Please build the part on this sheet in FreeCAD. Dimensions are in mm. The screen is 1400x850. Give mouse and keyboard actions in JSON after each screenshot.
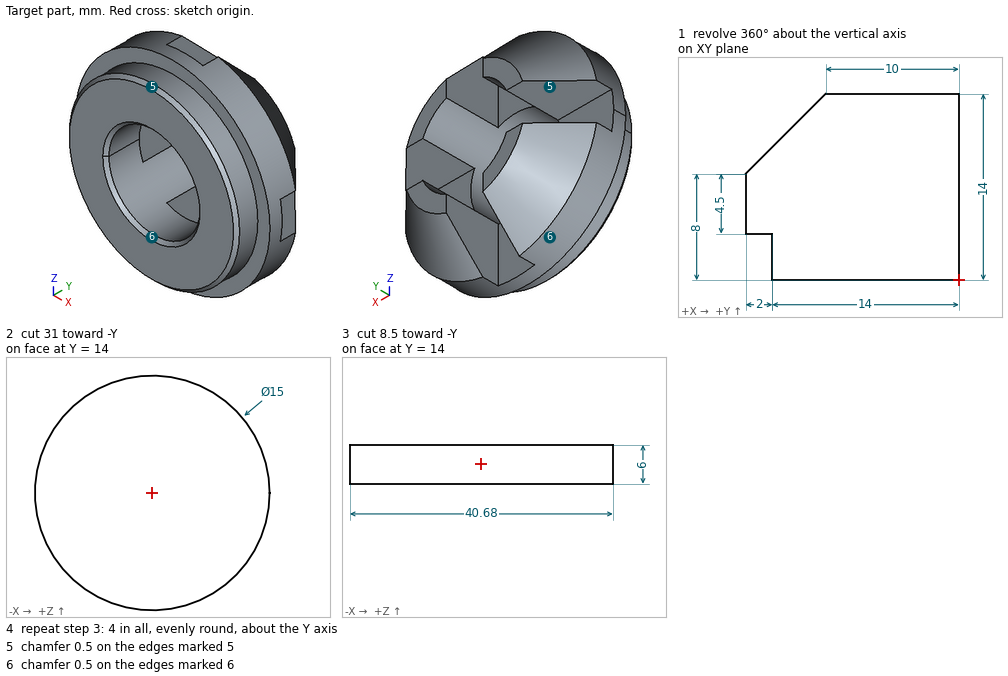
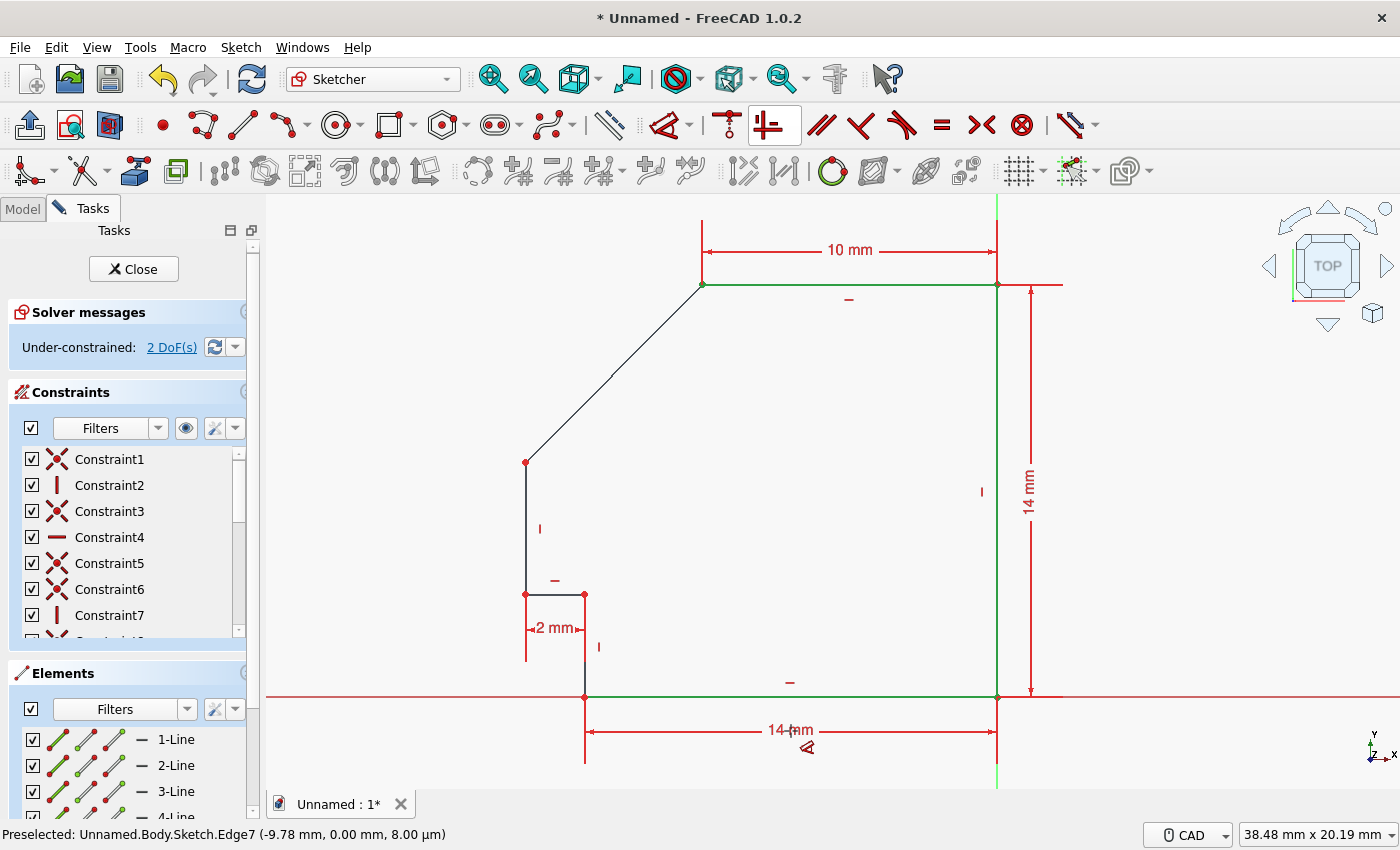
{"action": "left_click", "coordinate": [526, 463]}
{"action": "left_click", "coordinate": [1031, 580]}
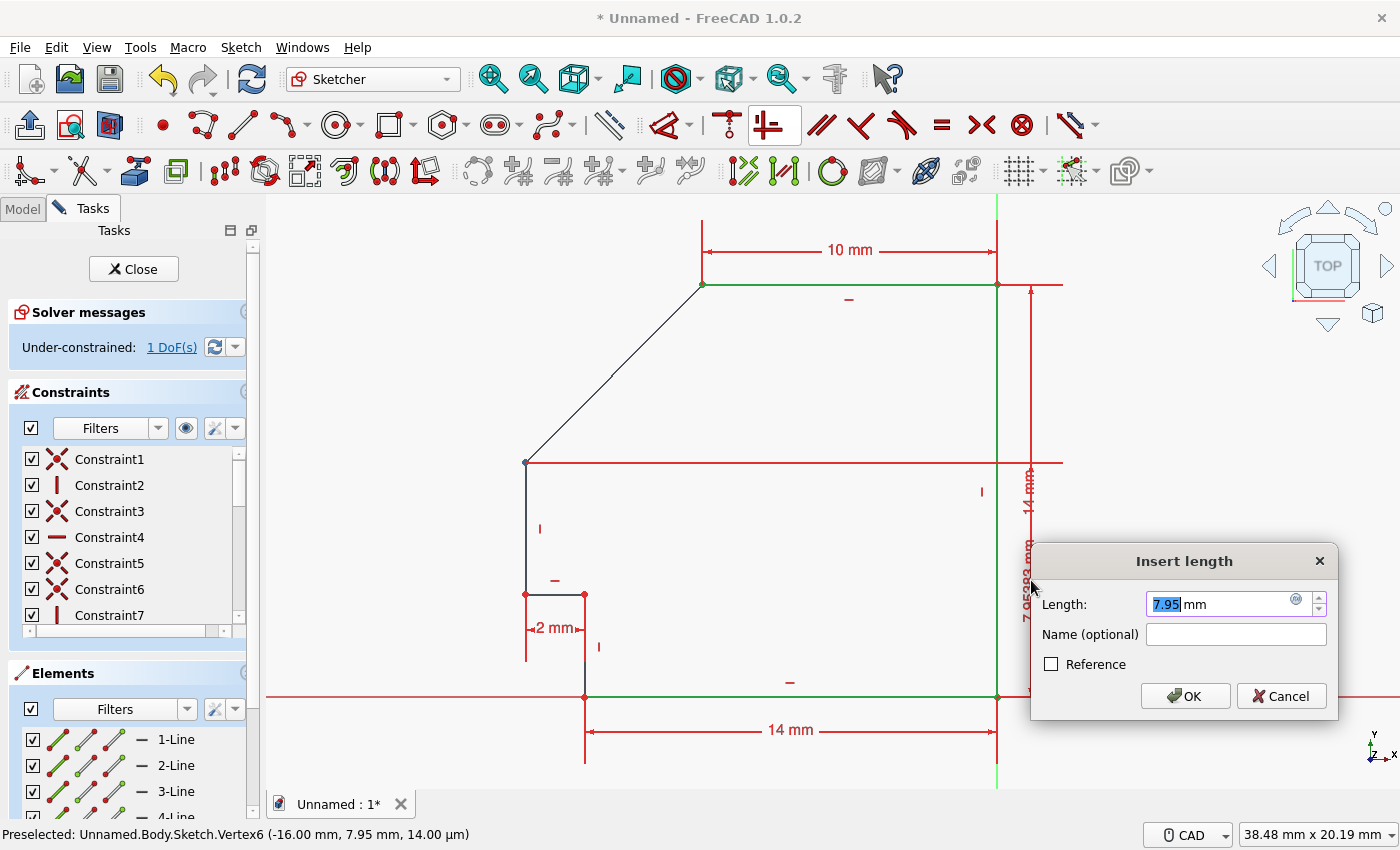
{"action": "type", "text": "8"}
{"action": "key", "text": "Return"}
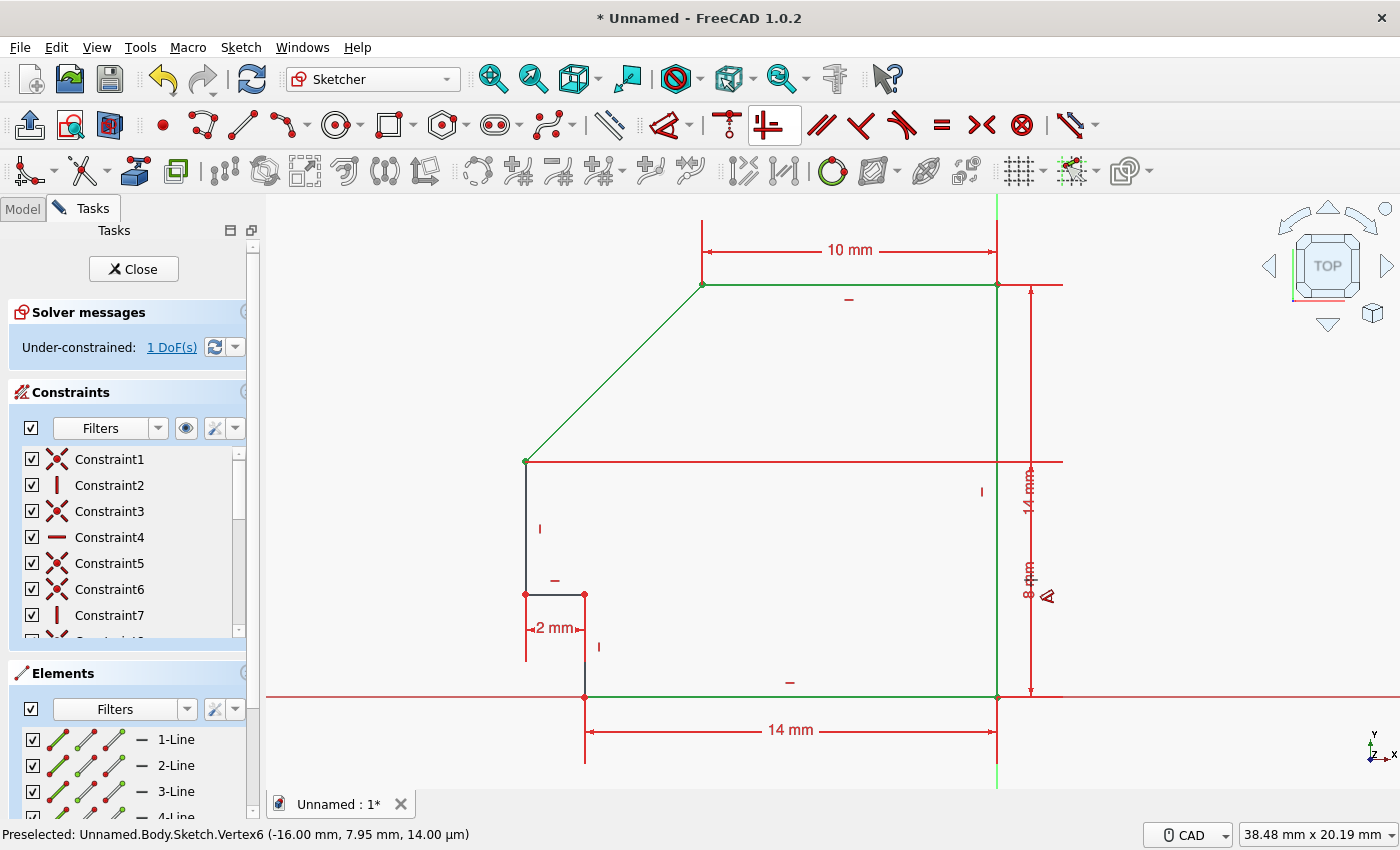
{"action": "left_click", "coordinate": [526, 502]}
{"action": "left_click", "coordinate": [492, 528]}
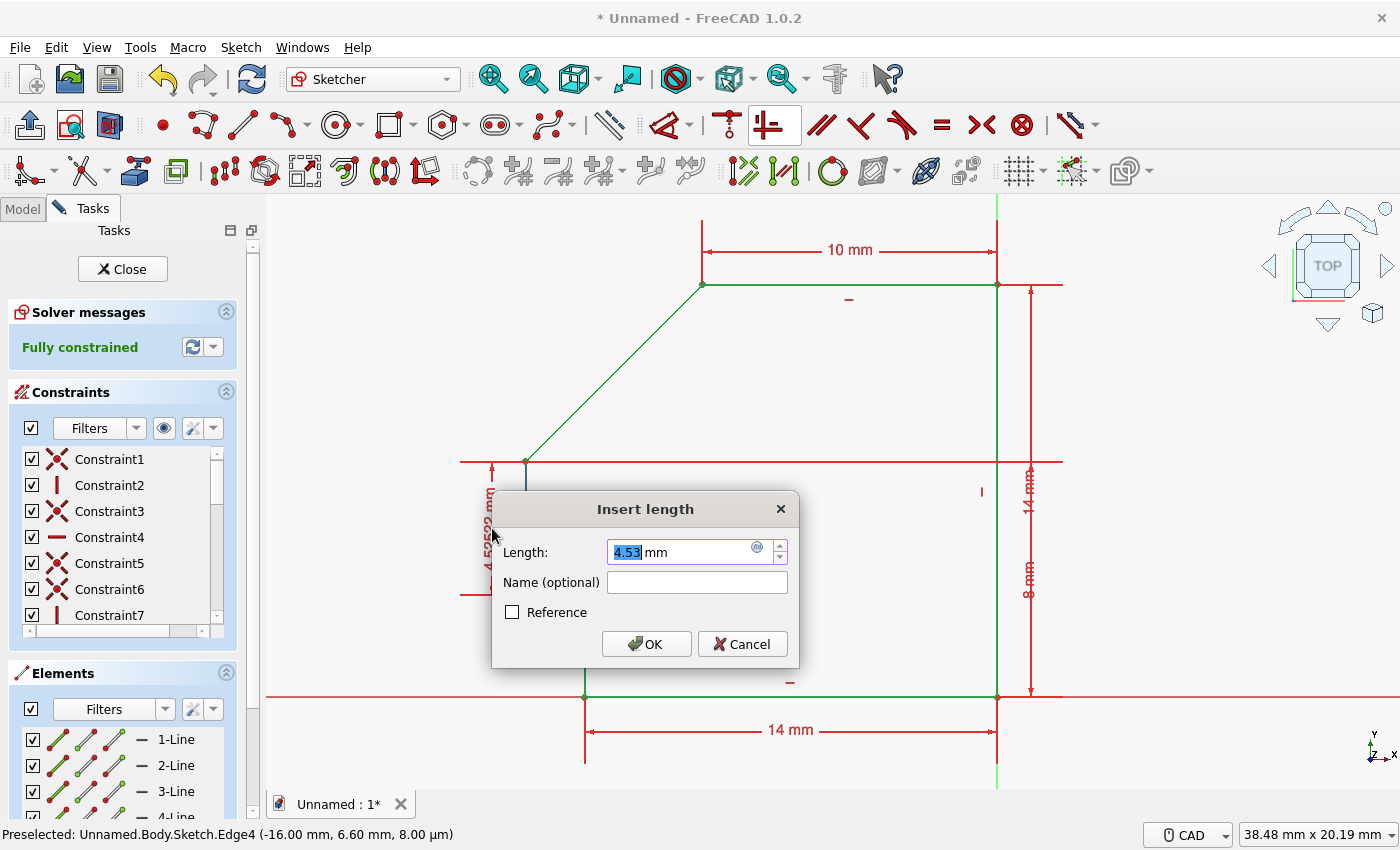
{"action": "type", "text": "4.5"}
{"action": "key", "text": "Return"}
{"action": "key", "text": "Escape"}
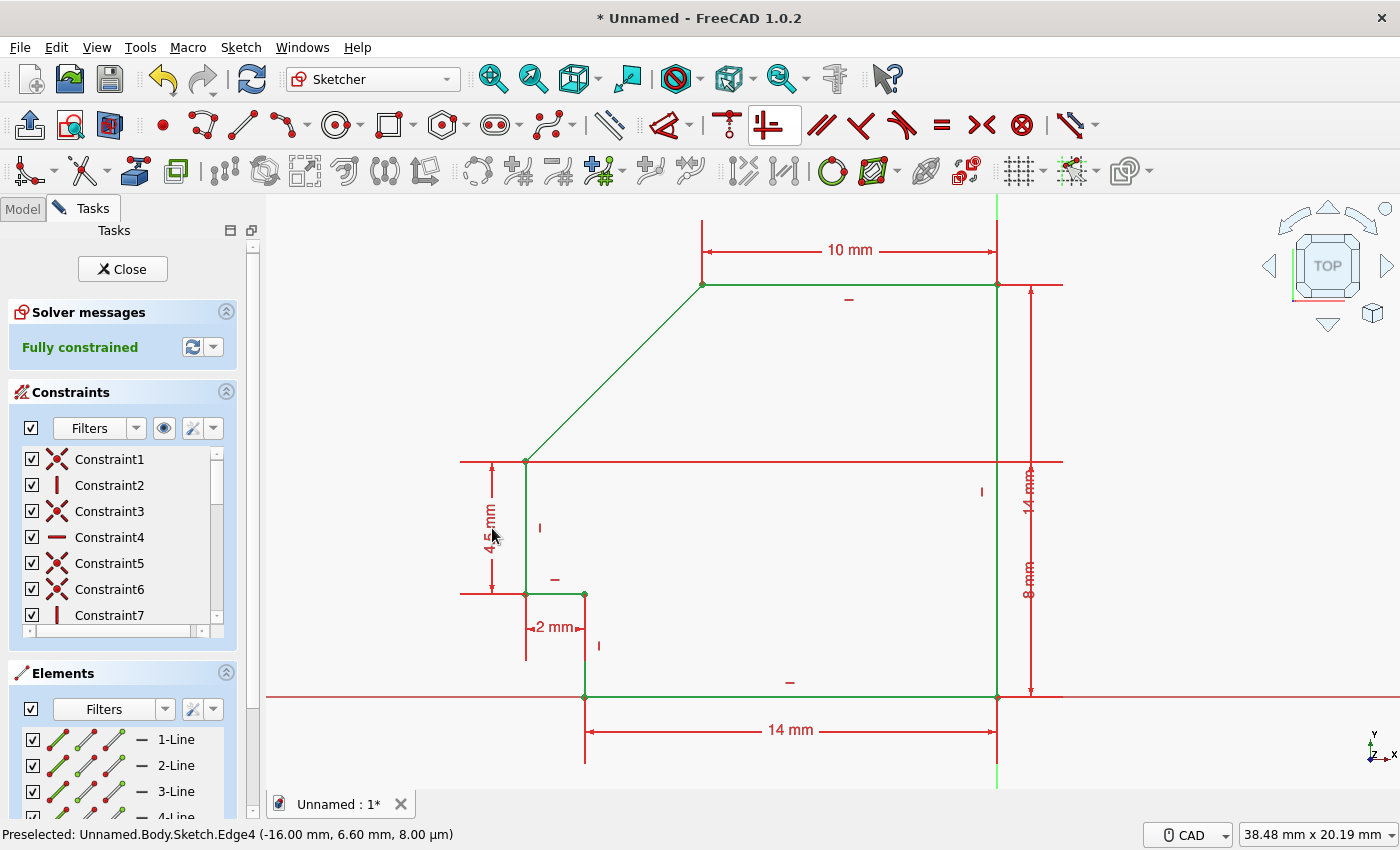
{"action": "left_click", "coordinate": [123, 269]}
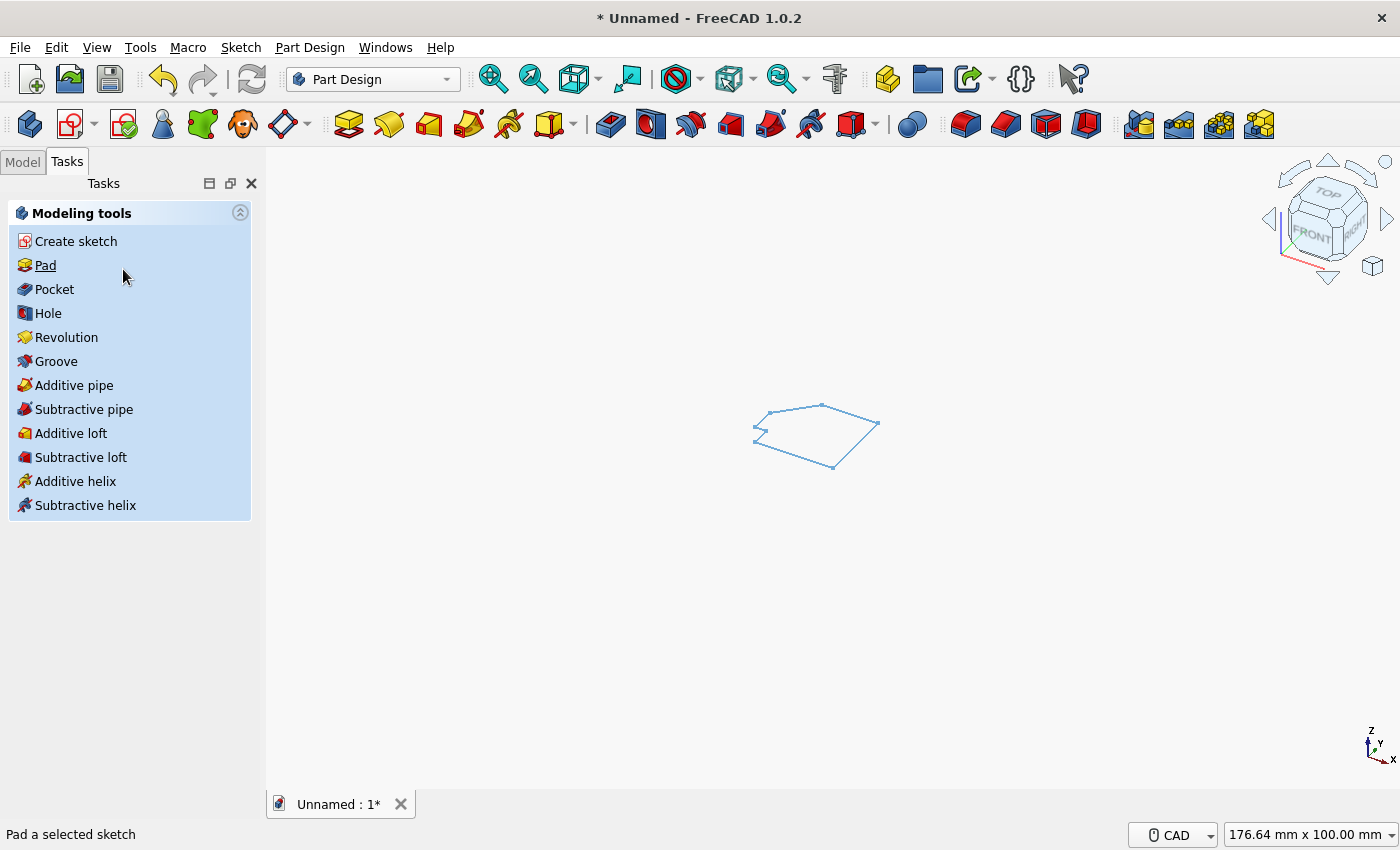
{"action": "left_click", "coordinate": [390, 124]}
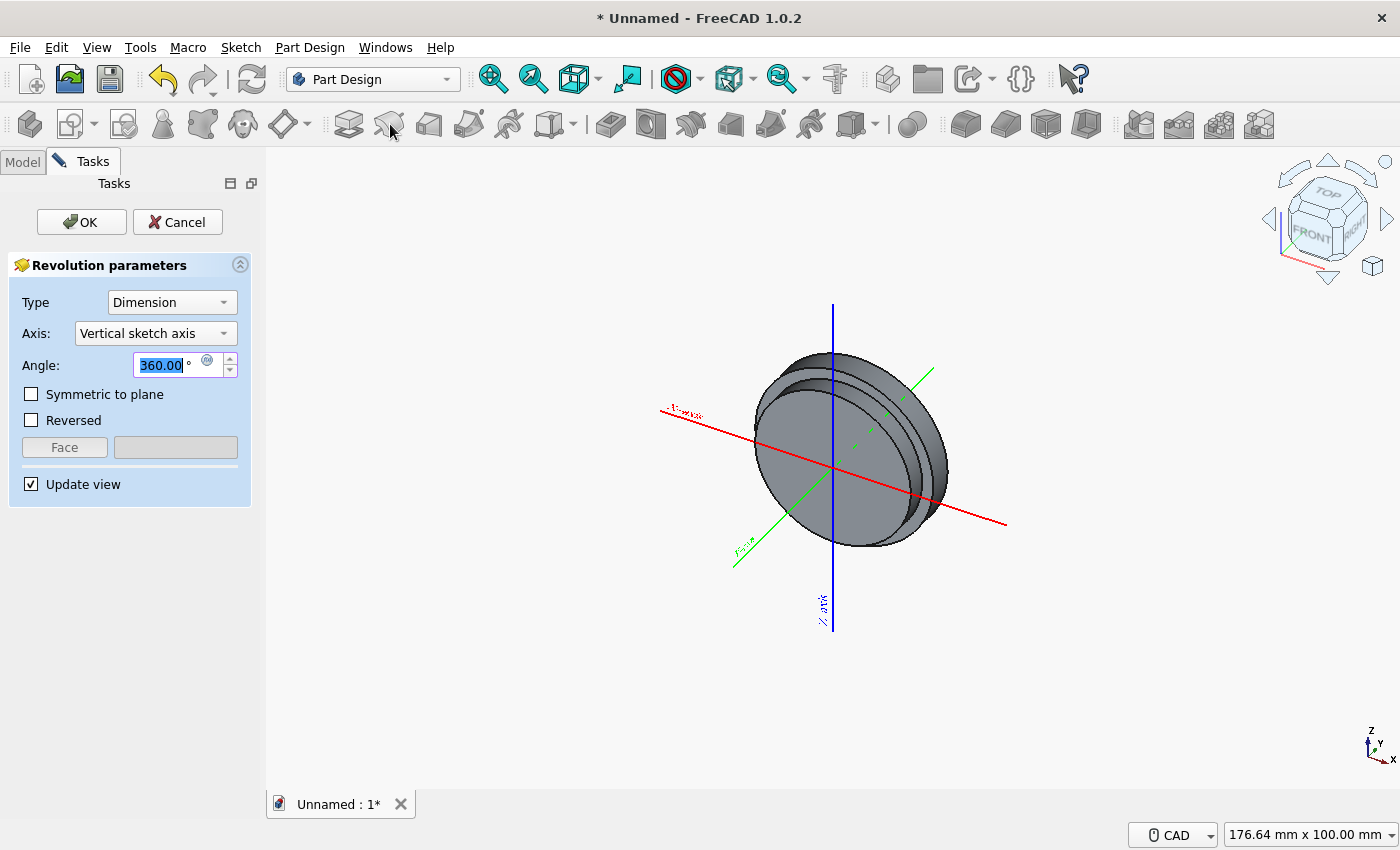
{"action": "left_click", "coordinate": [82, 222]}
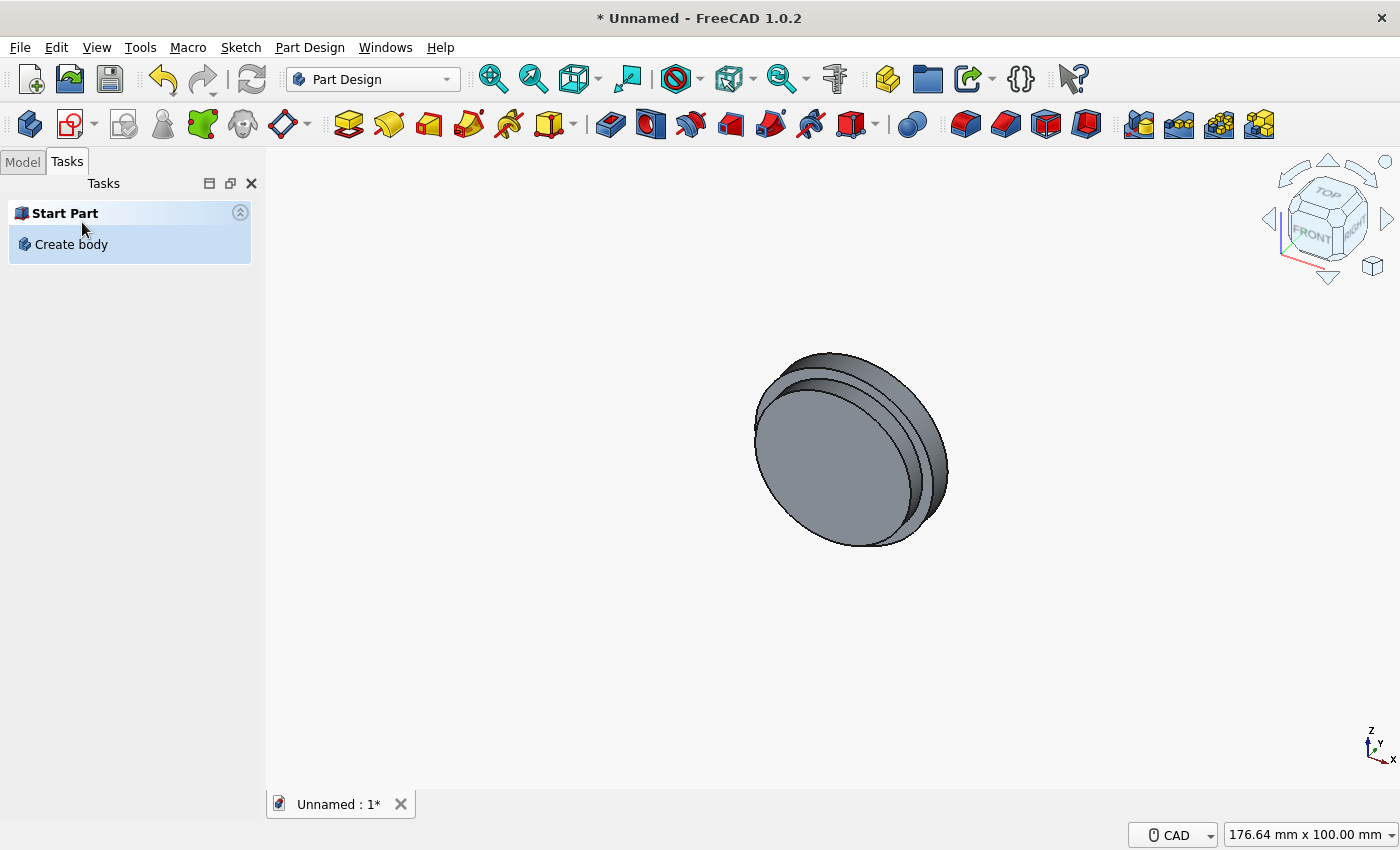
{"action": "left_click", "coordinate": [494, 80]}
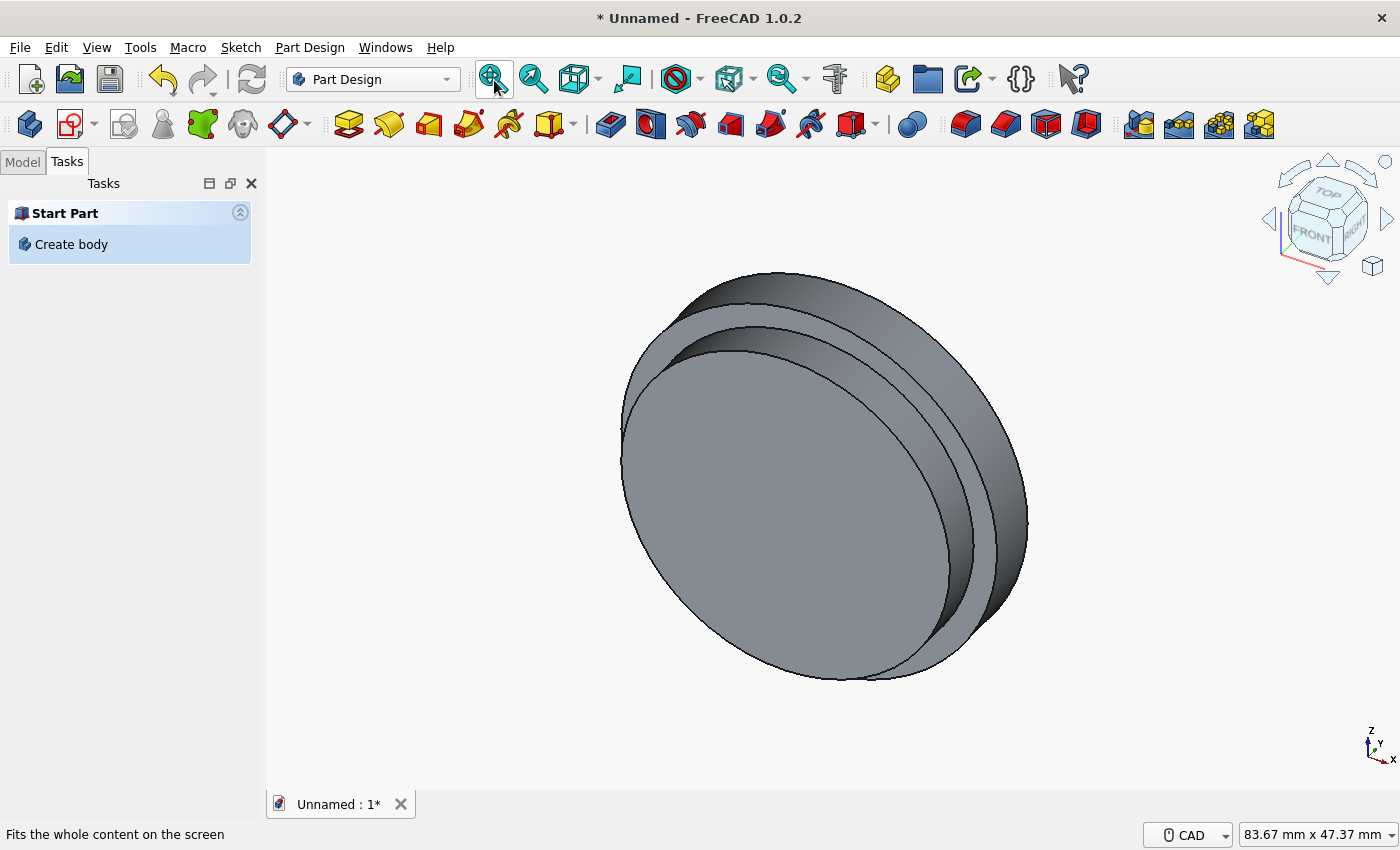
{"action": "key", "text": "4"}